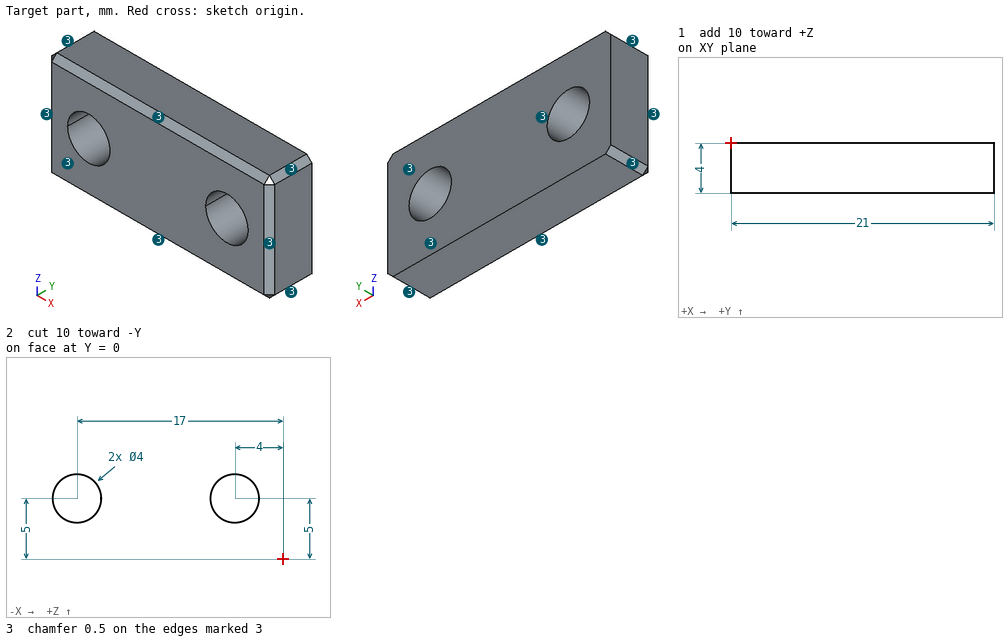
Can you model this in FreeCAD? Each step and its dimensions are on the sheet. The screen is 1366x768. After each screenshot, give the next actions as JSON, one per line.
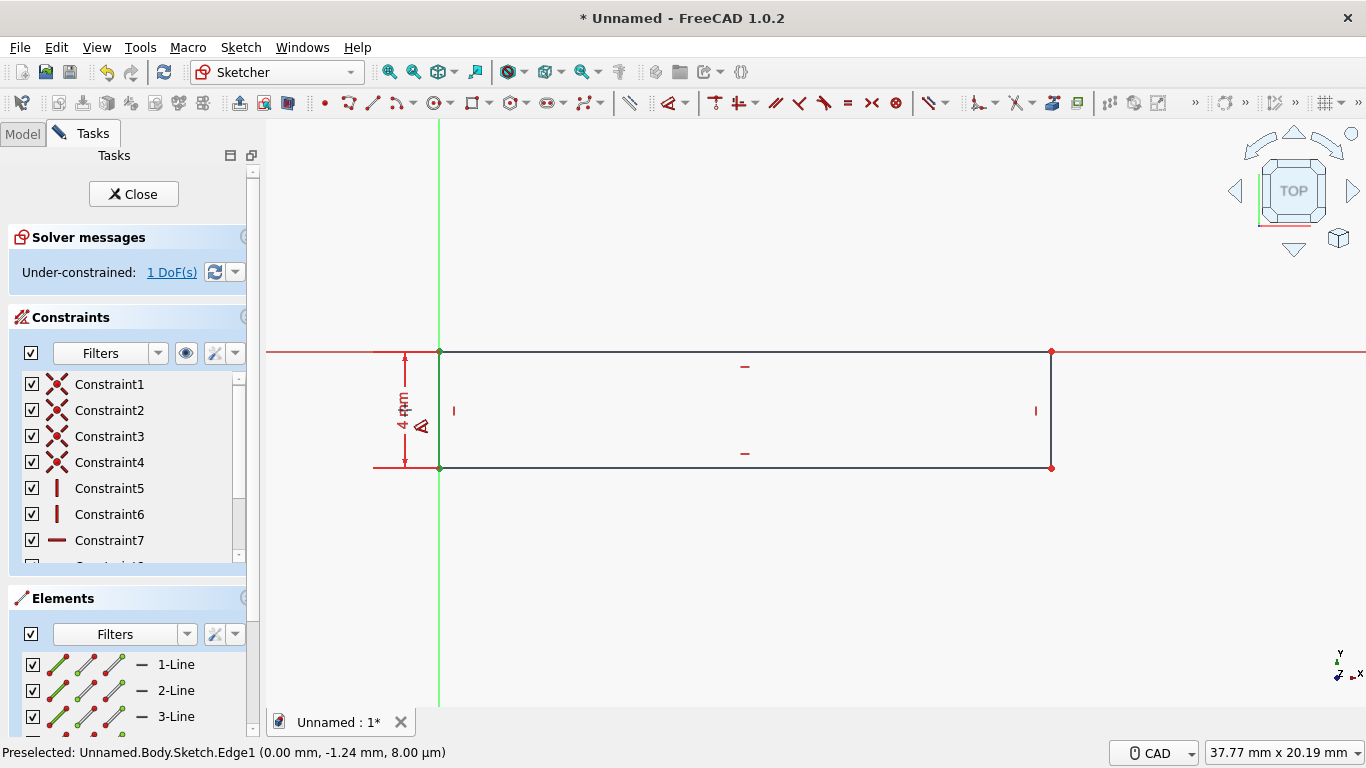
{"action": "left_click", "coordinate": [623, 468]}
{"action": "left_click", "coordinate": [745, 502]}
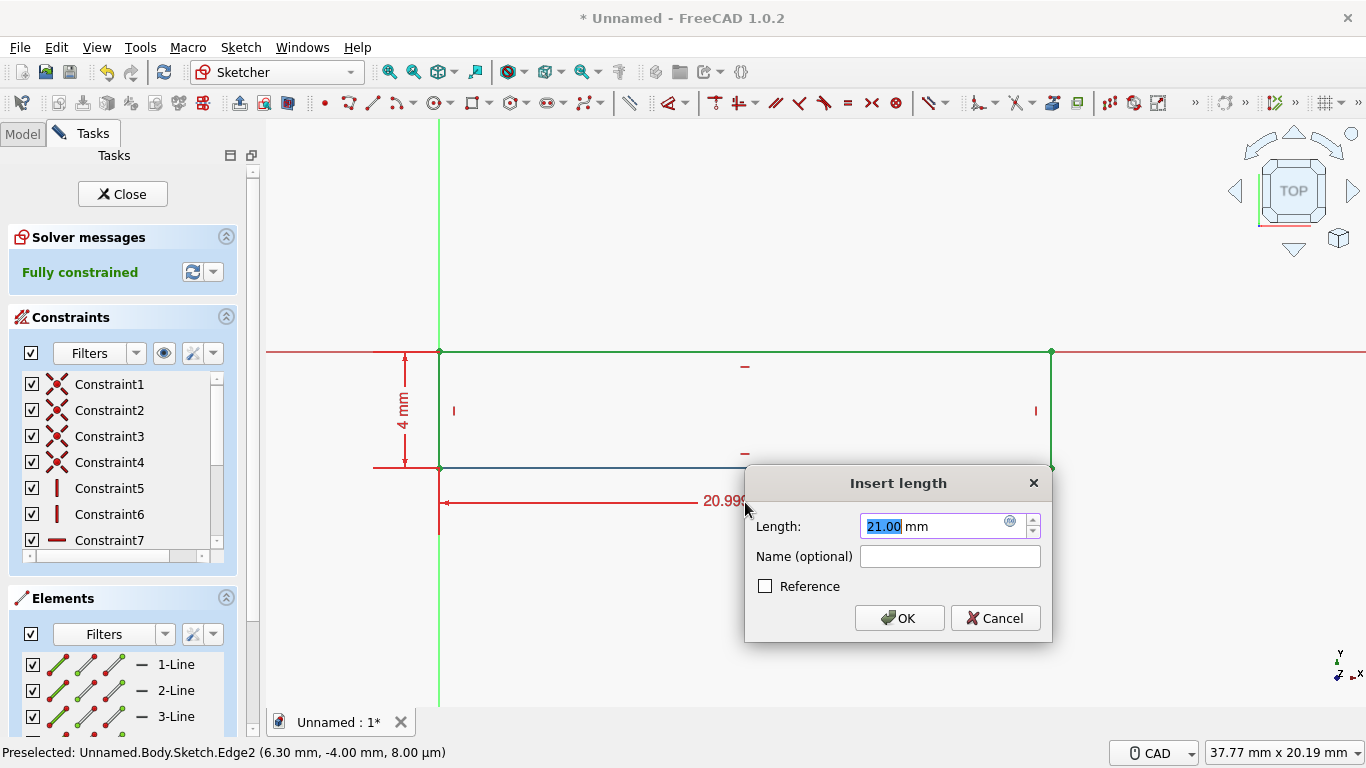
{"action": "type", "text": "21"}
{"action": "key", "text": "Return"}
{"action": "key", "text": "Escape"}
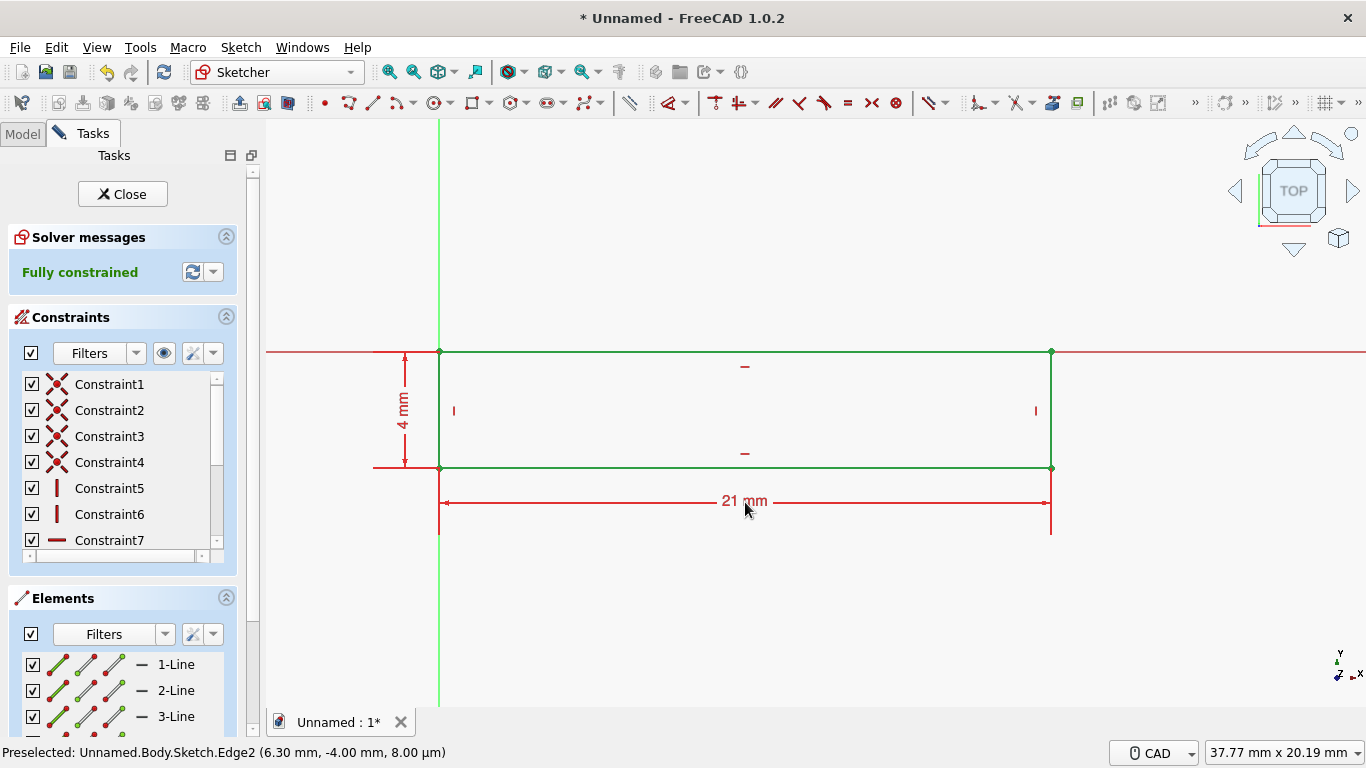
{"action": "left_click", "coordinate": [123, 194]}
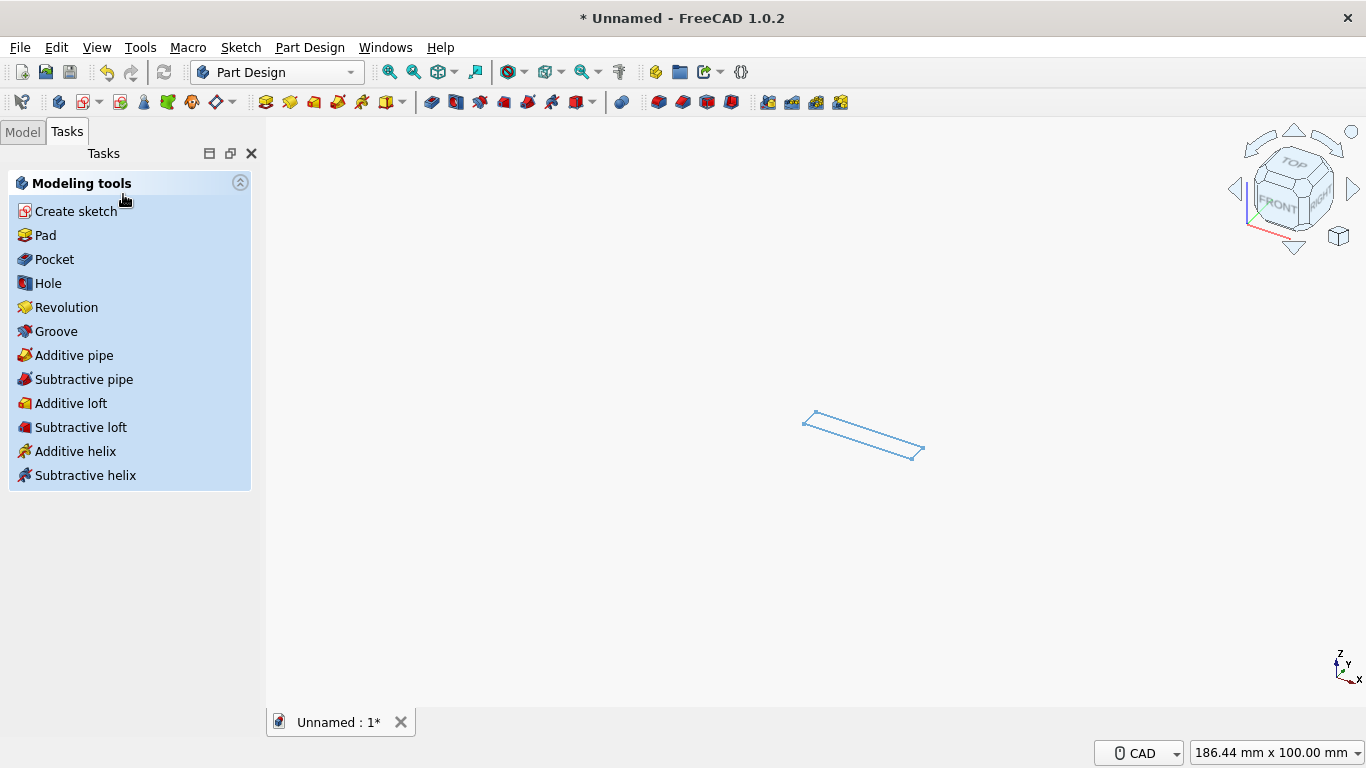
{"action": "left_click", "coordinate": [266, 102]}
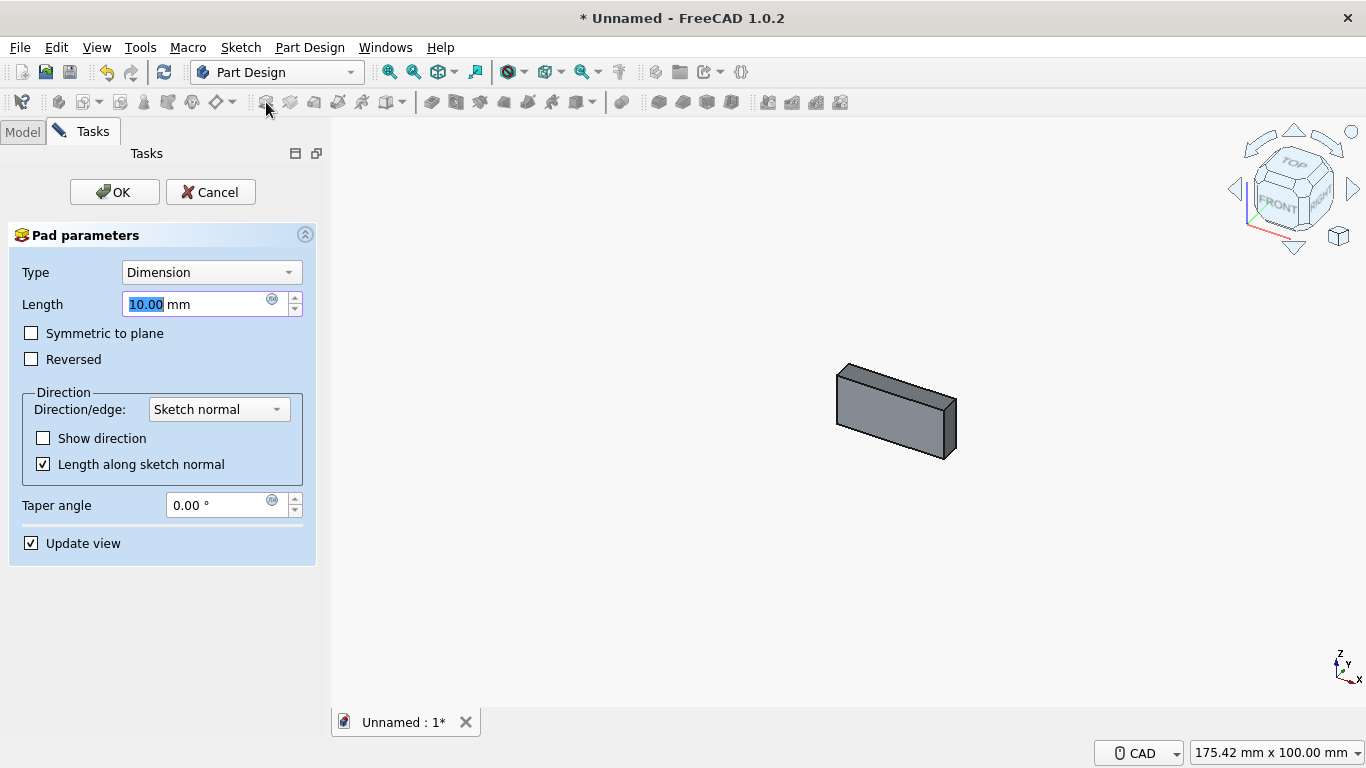
{"action": "type", "text": "10"}
{"action": "key", "text": "Tab"}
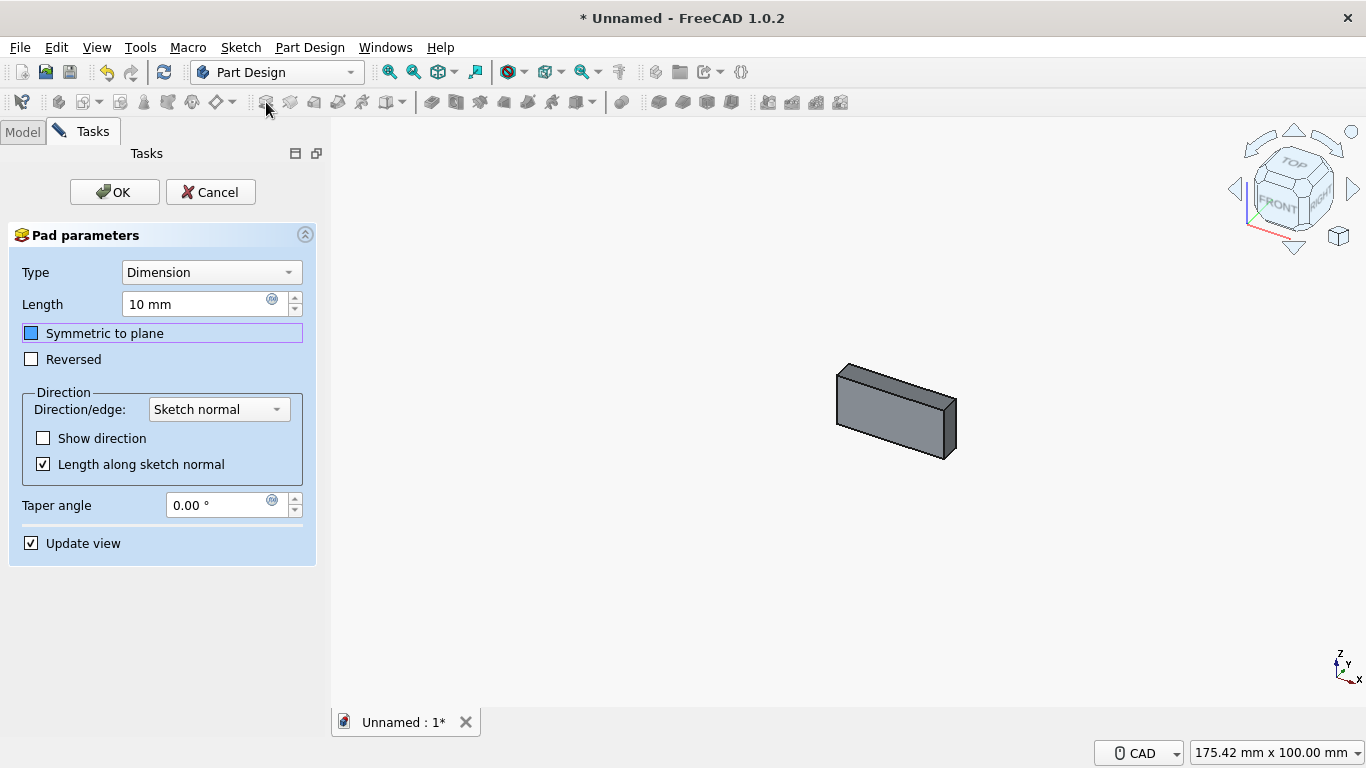
{"action": "left_click", "coordinate": [115, 192]}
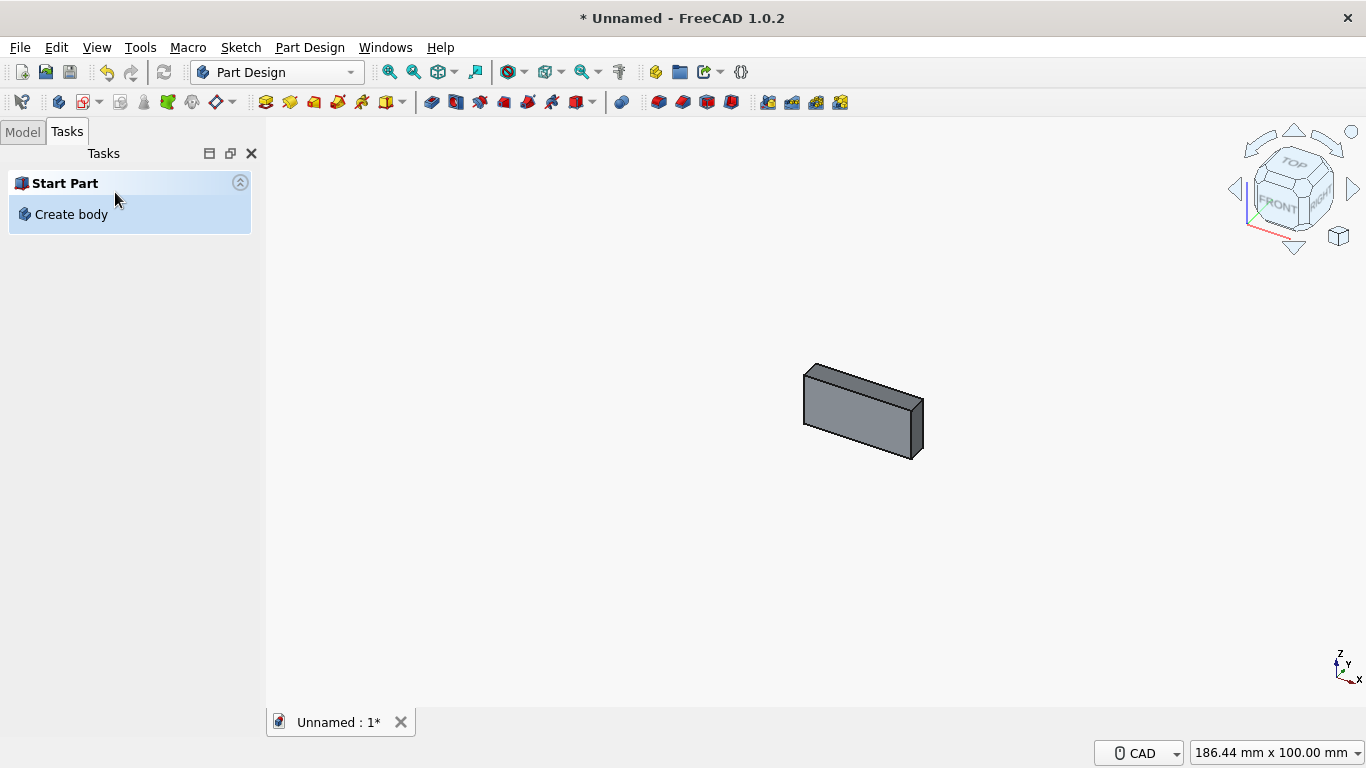
{"action": "left_click", "coordinate": [390, 72]}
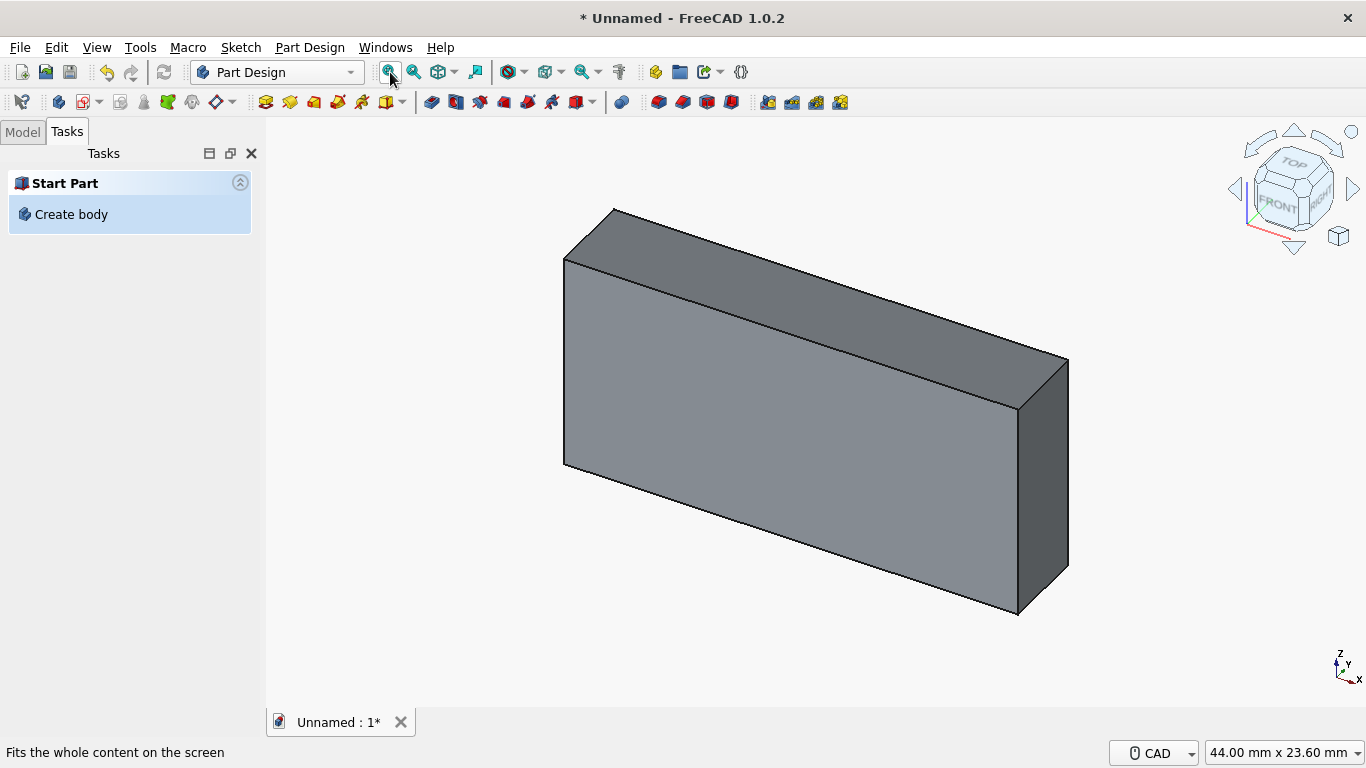
{"action": "key", "text": "4"}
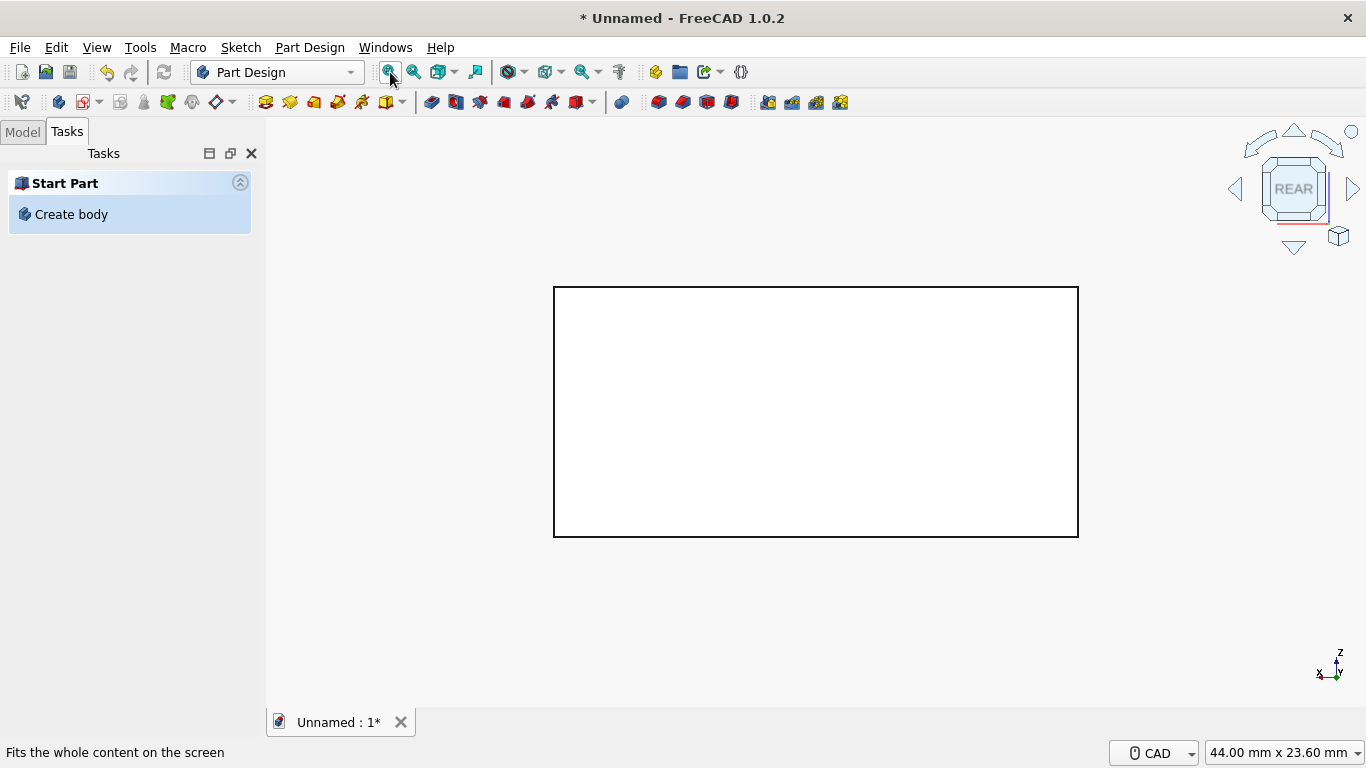
{"action": "left_click", "coordinate": [741, 411]}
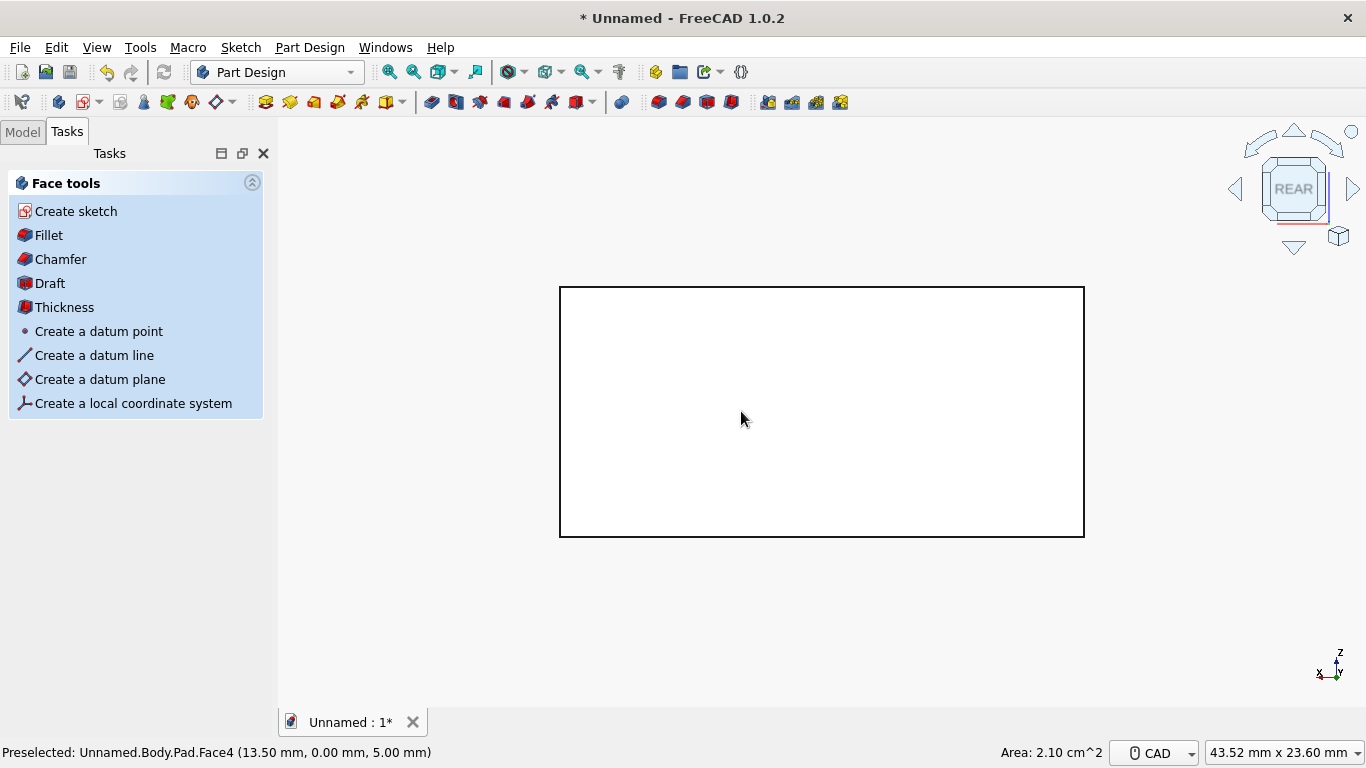
{"action": "left_click", "coordinate": [84, 102]}